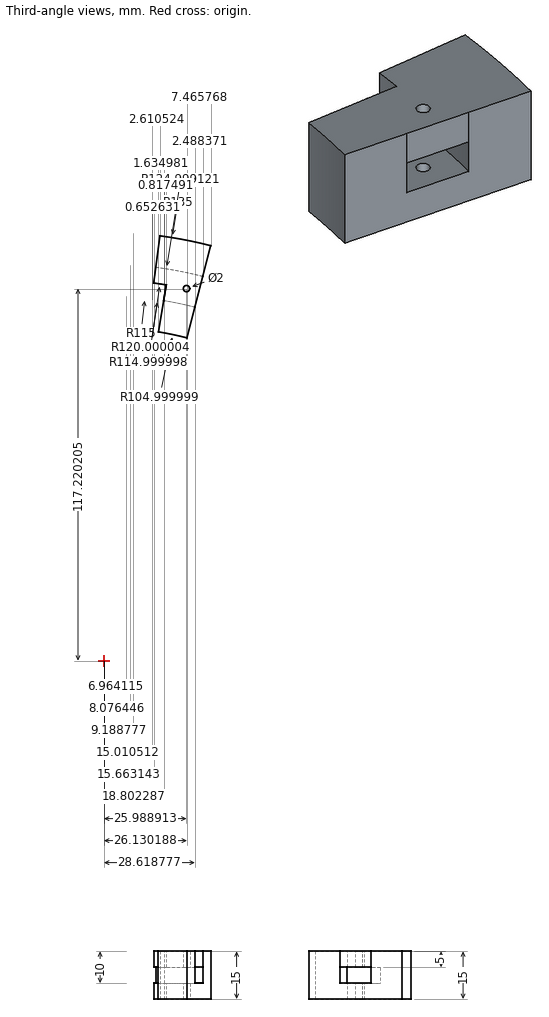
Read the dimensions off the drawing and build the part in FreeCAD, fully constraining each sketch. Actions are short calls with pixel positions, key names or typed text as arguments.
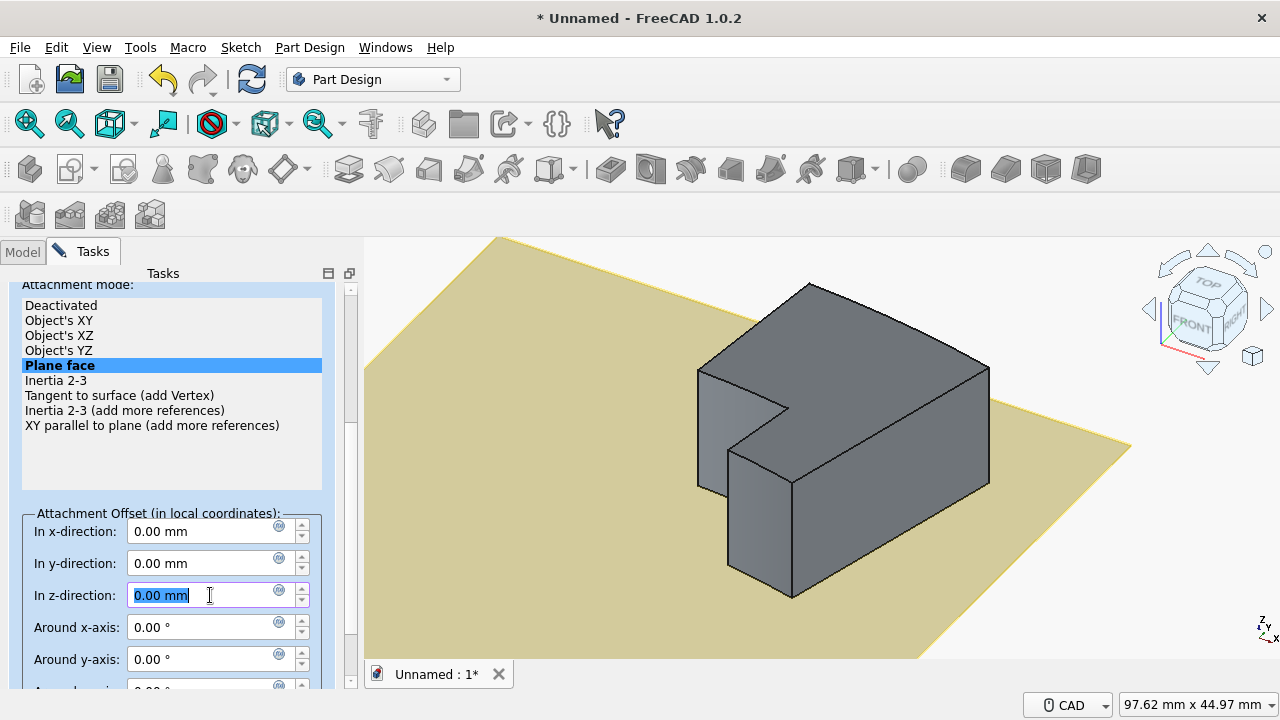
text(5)
key(Tab)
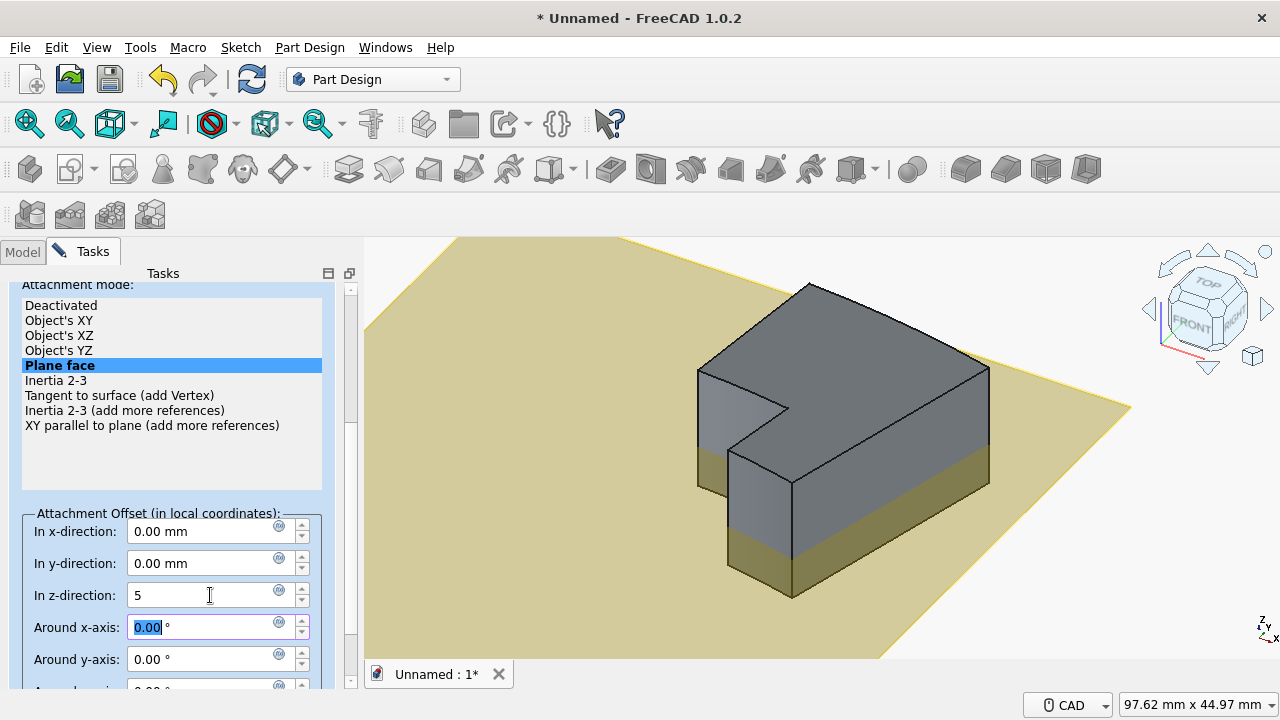
scroll(351, 486, up, 5)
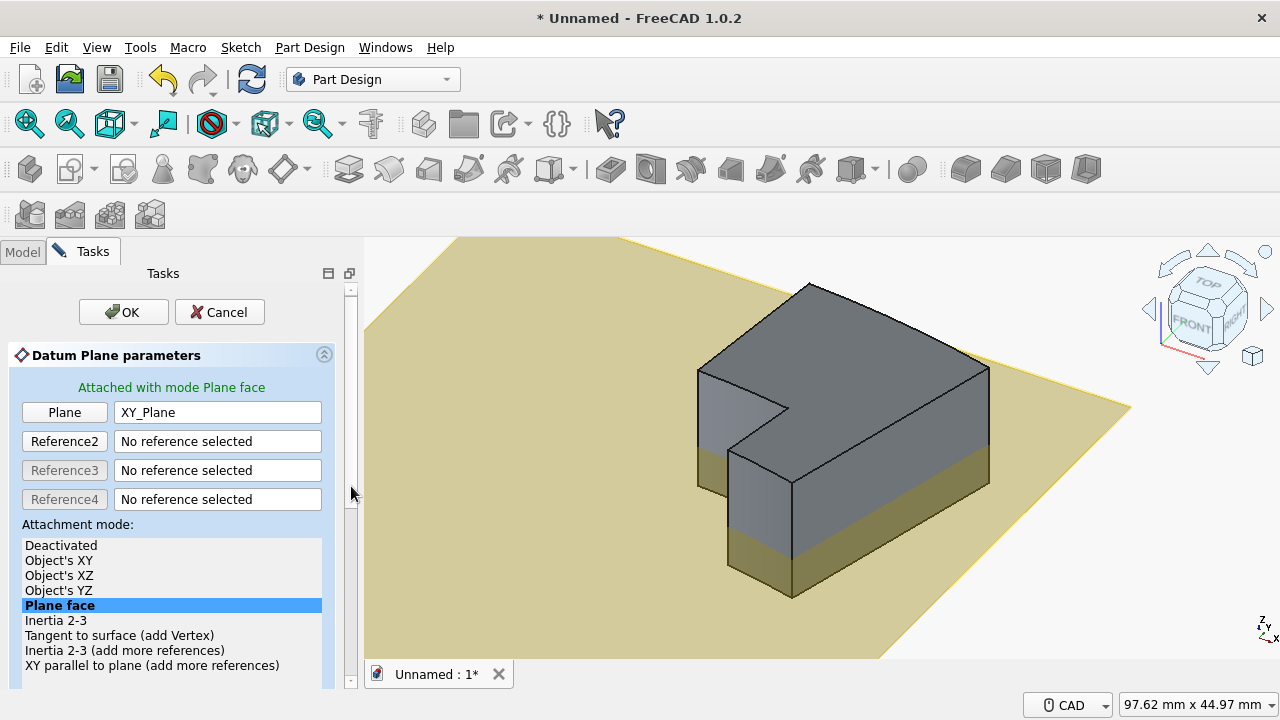
click(124, 312)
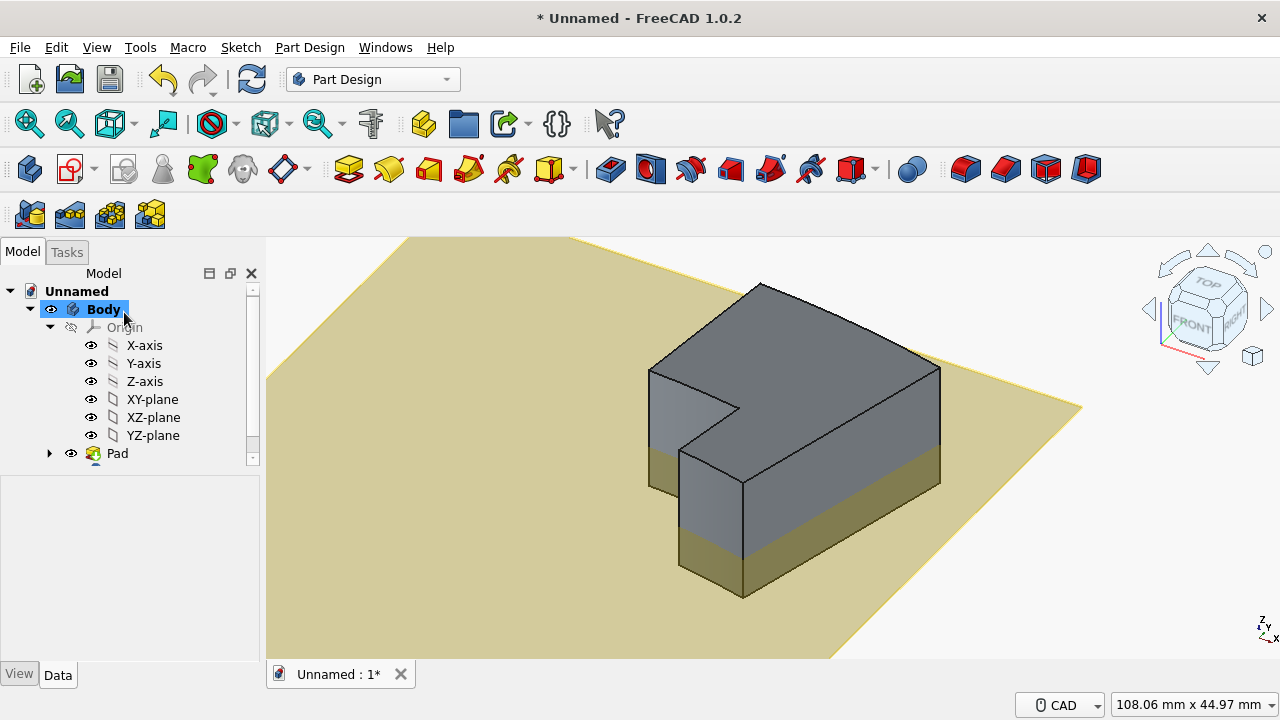
scroll(100, 377, down, 3)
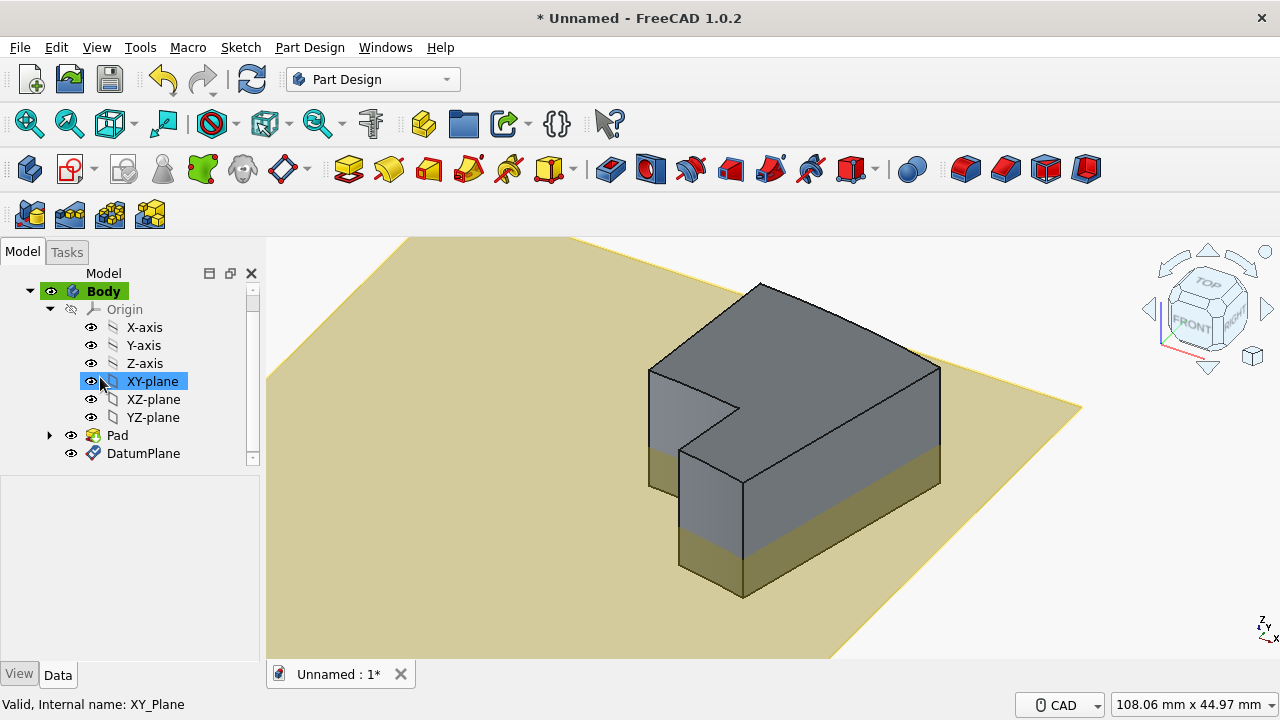
click(116, 453)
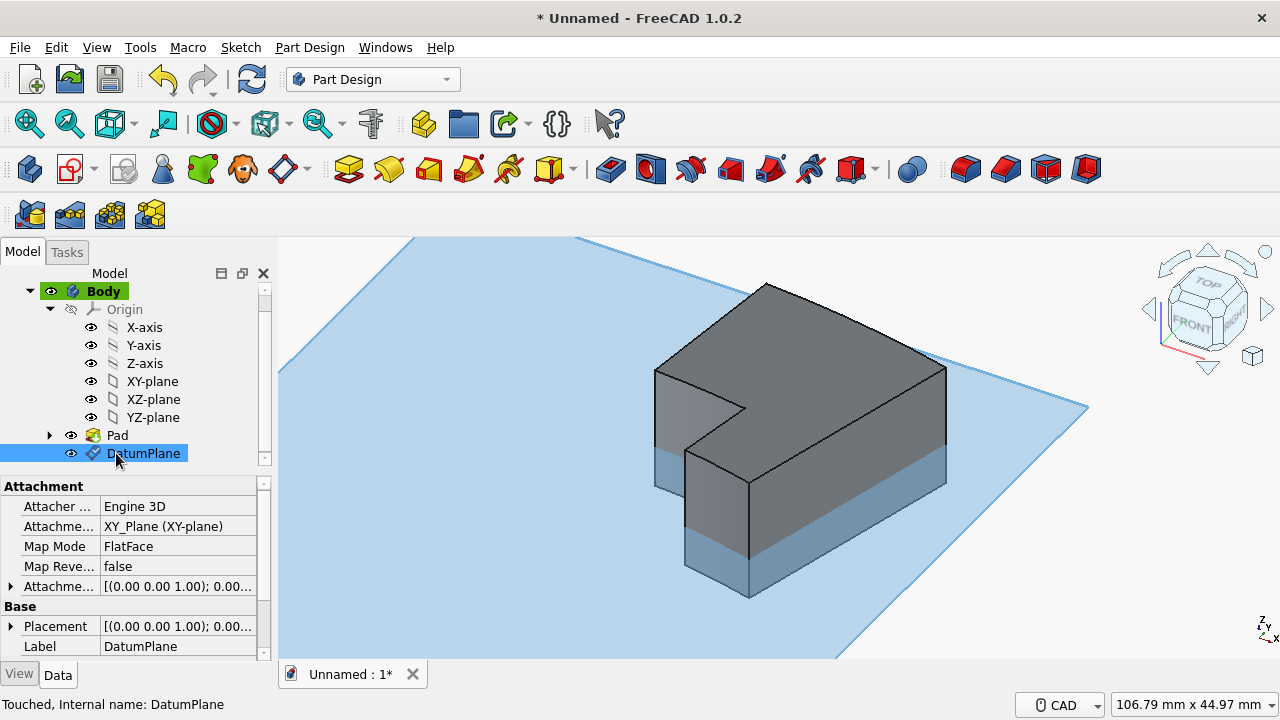
click(70, 170)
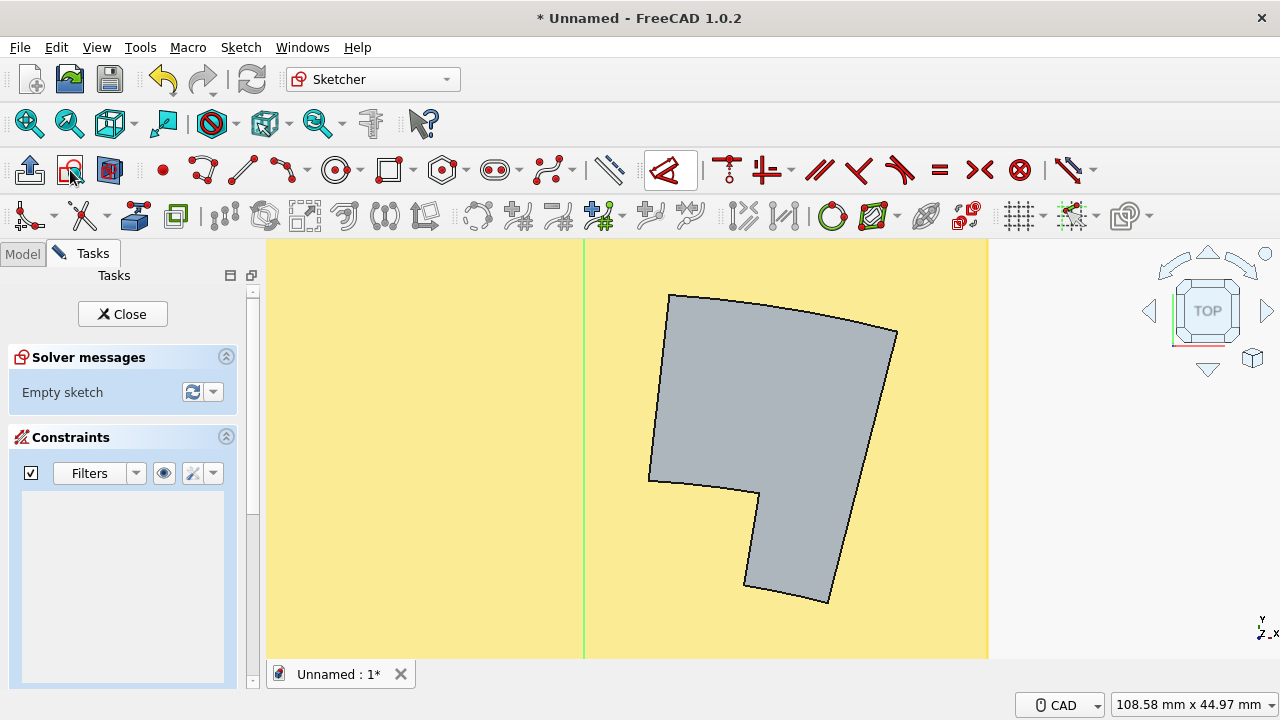
click(110, 170)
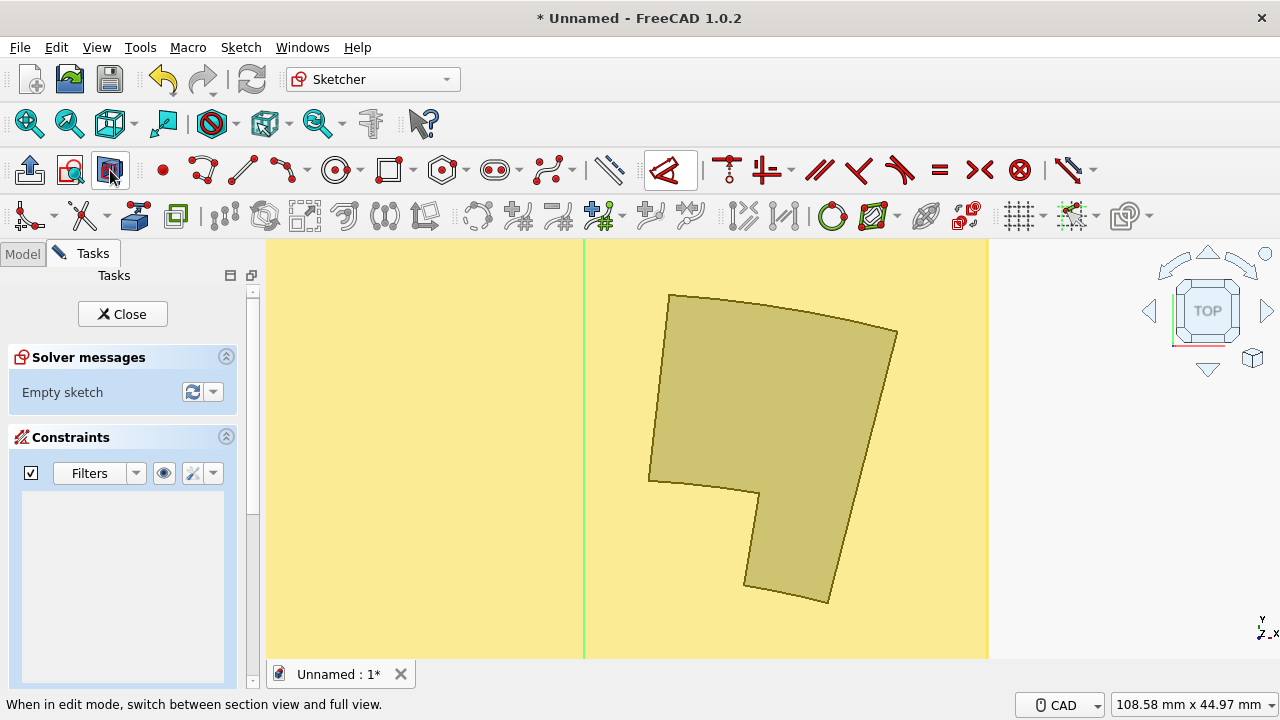
scroll(808, 451, up, 4)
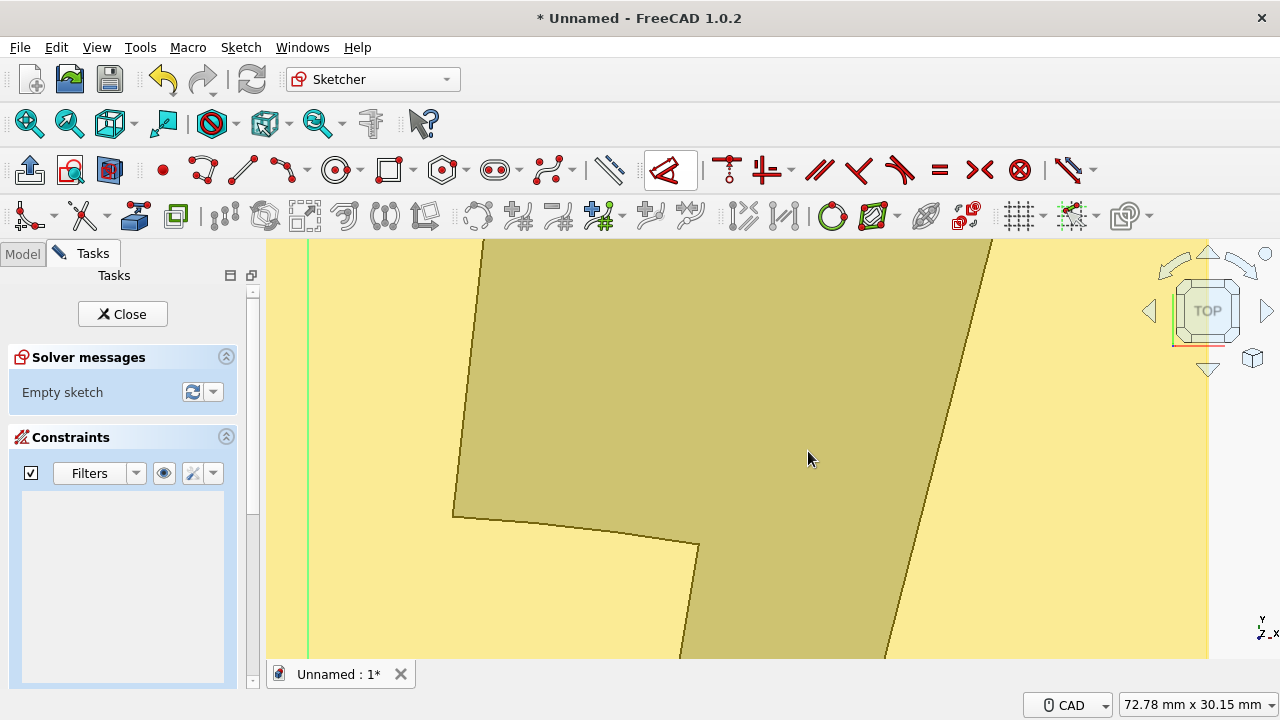
click(244, 170)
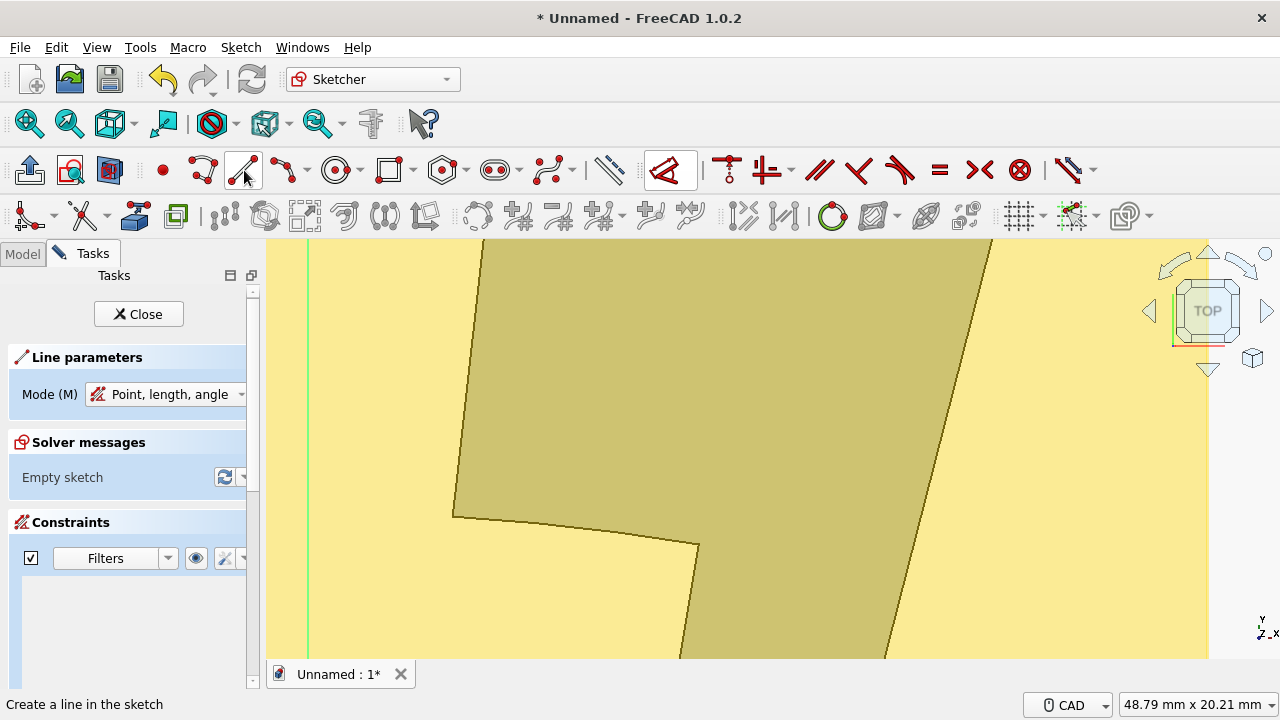
click(903, 587)
click(954, 386)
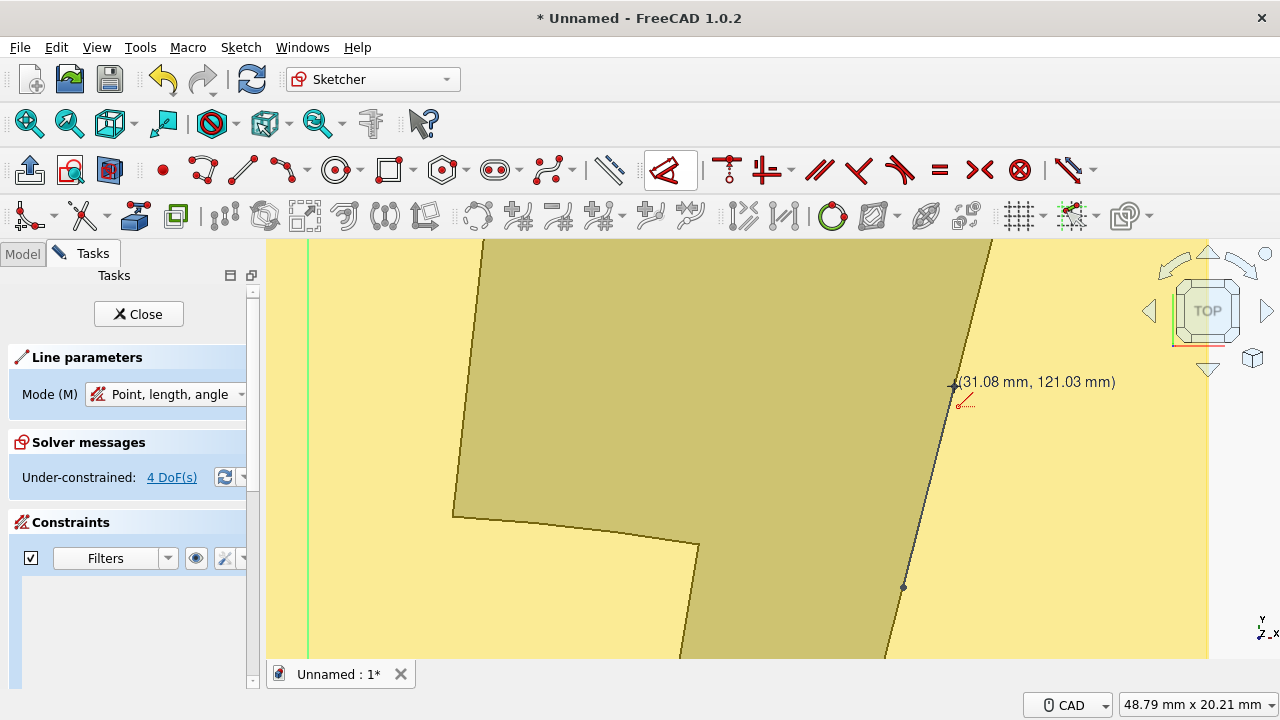
click(476, 310)
click(453, 517)